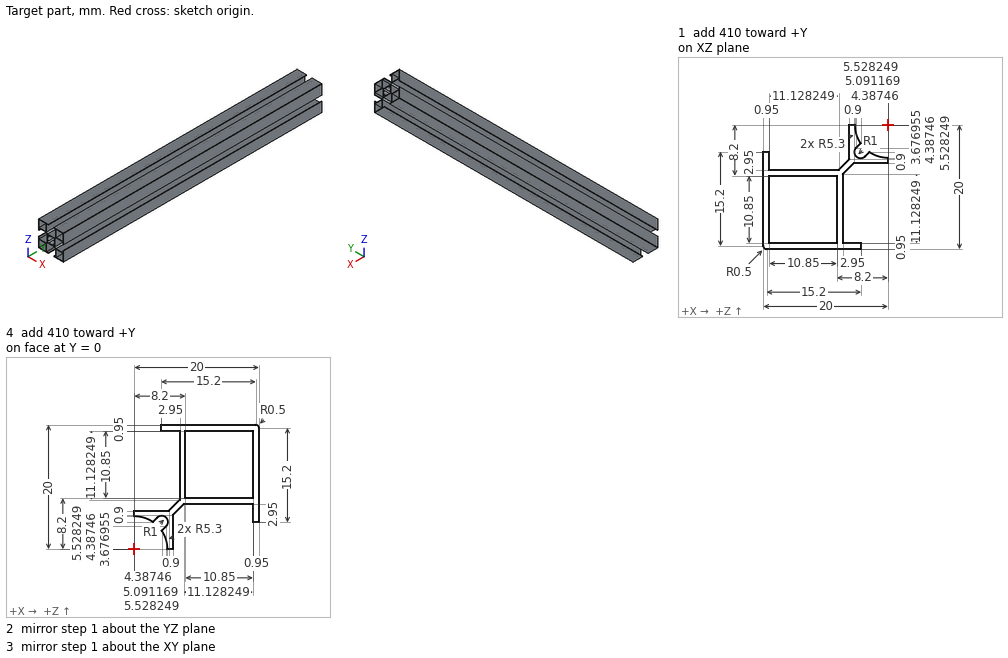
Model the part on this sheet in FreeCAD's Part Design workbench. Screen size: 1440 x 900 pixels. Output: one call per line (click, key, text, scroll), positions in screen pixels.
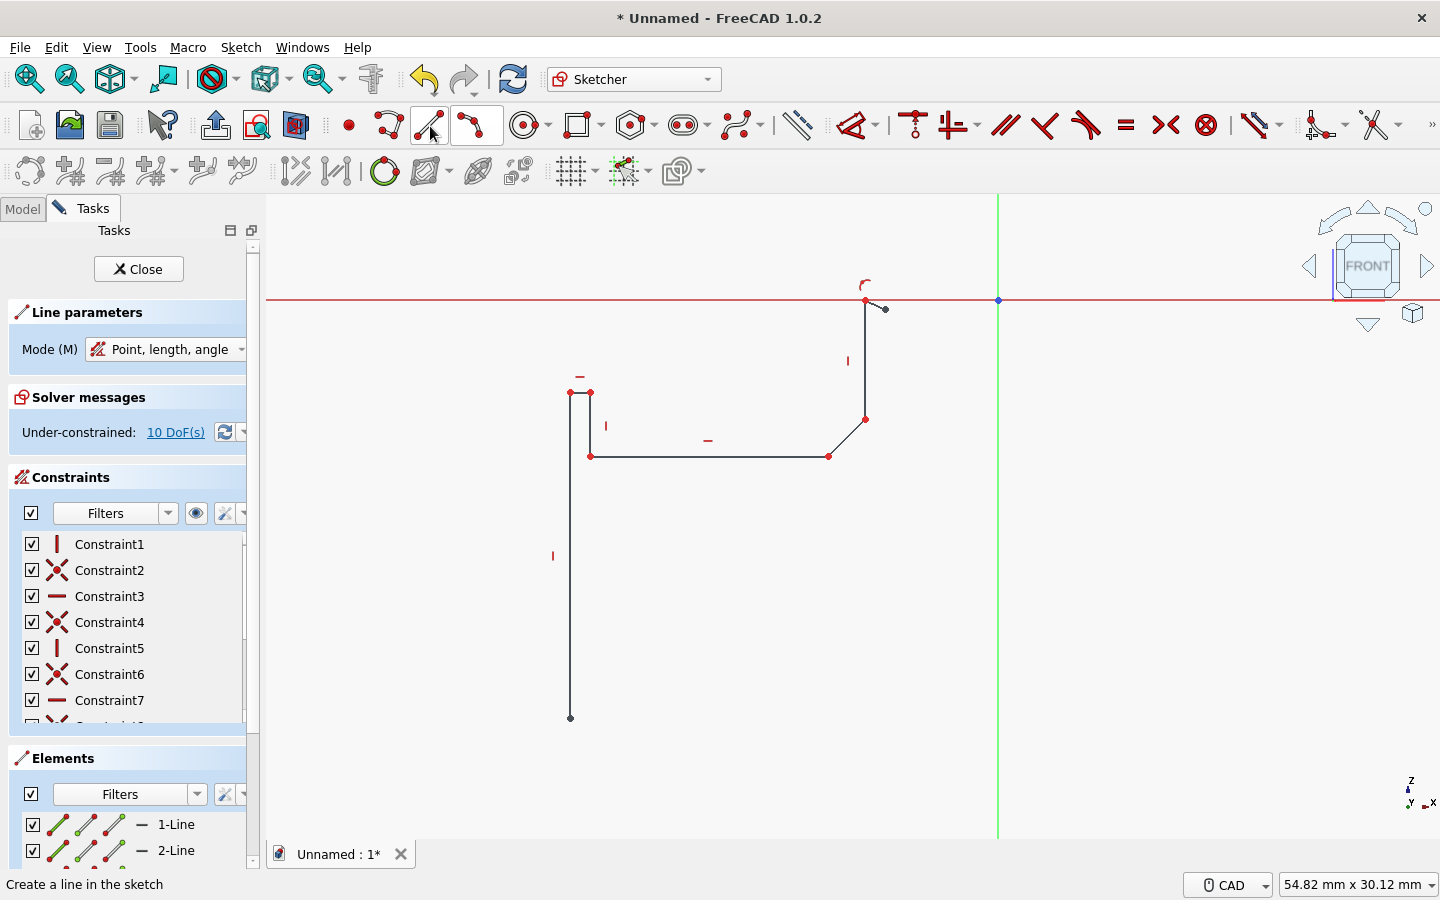
click(904, 364)
click(889, 379)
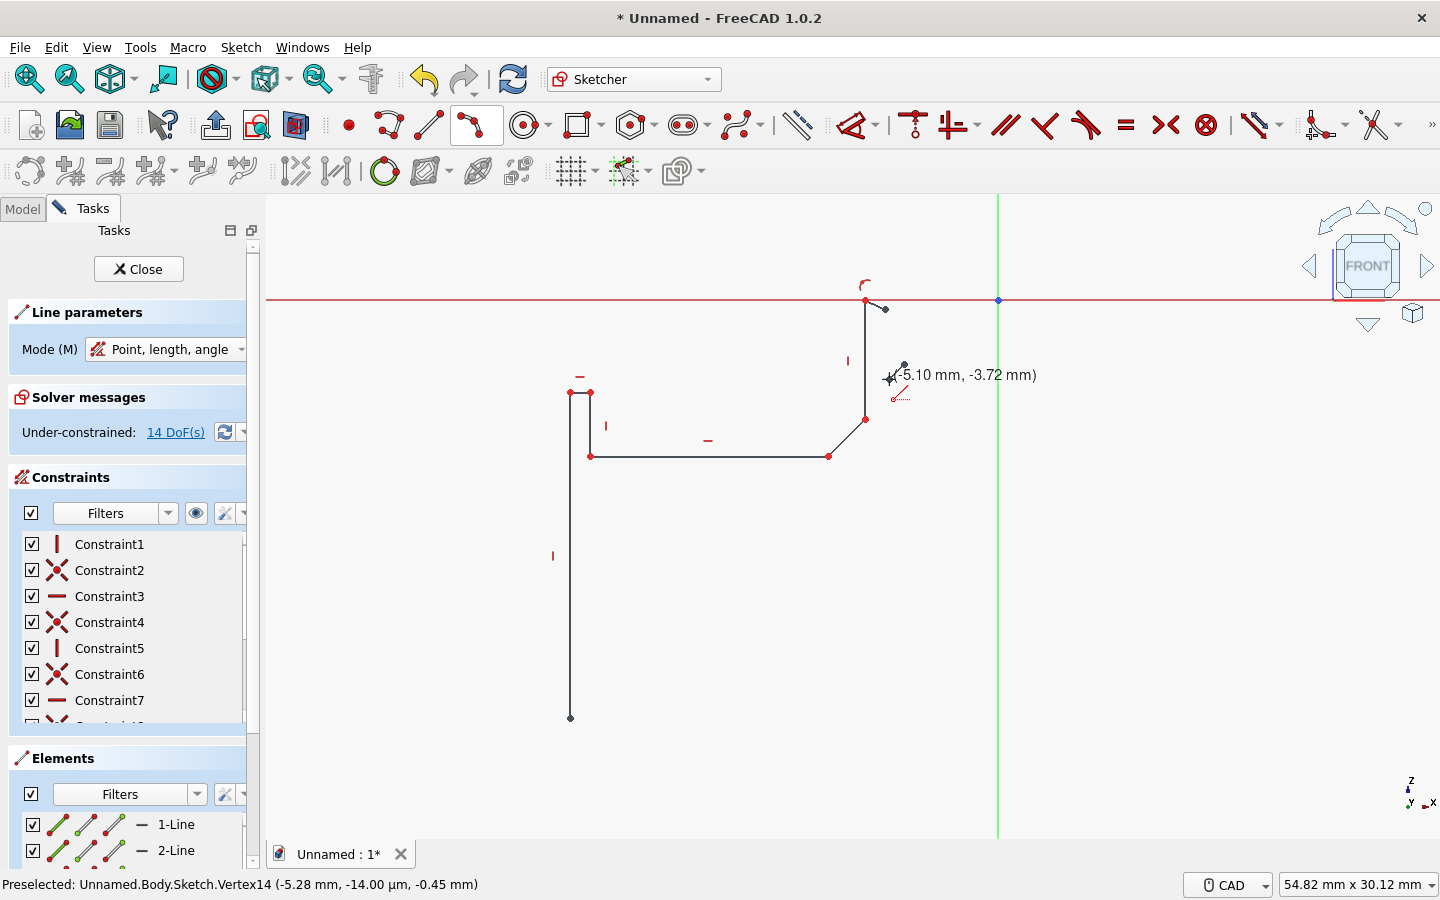
click(919, 409)
click(934, 394)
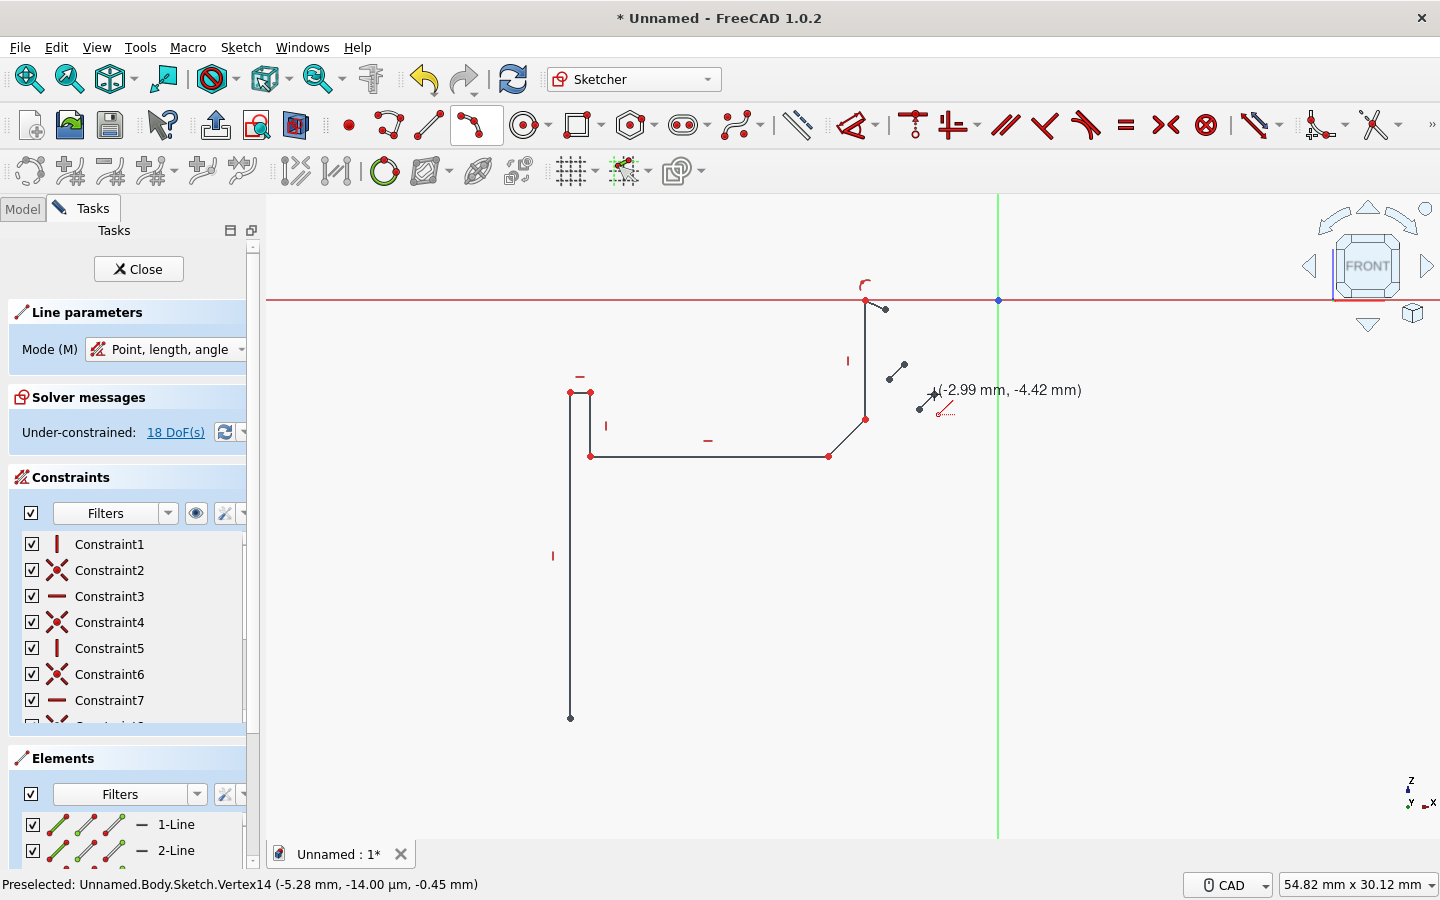
click(390, 126)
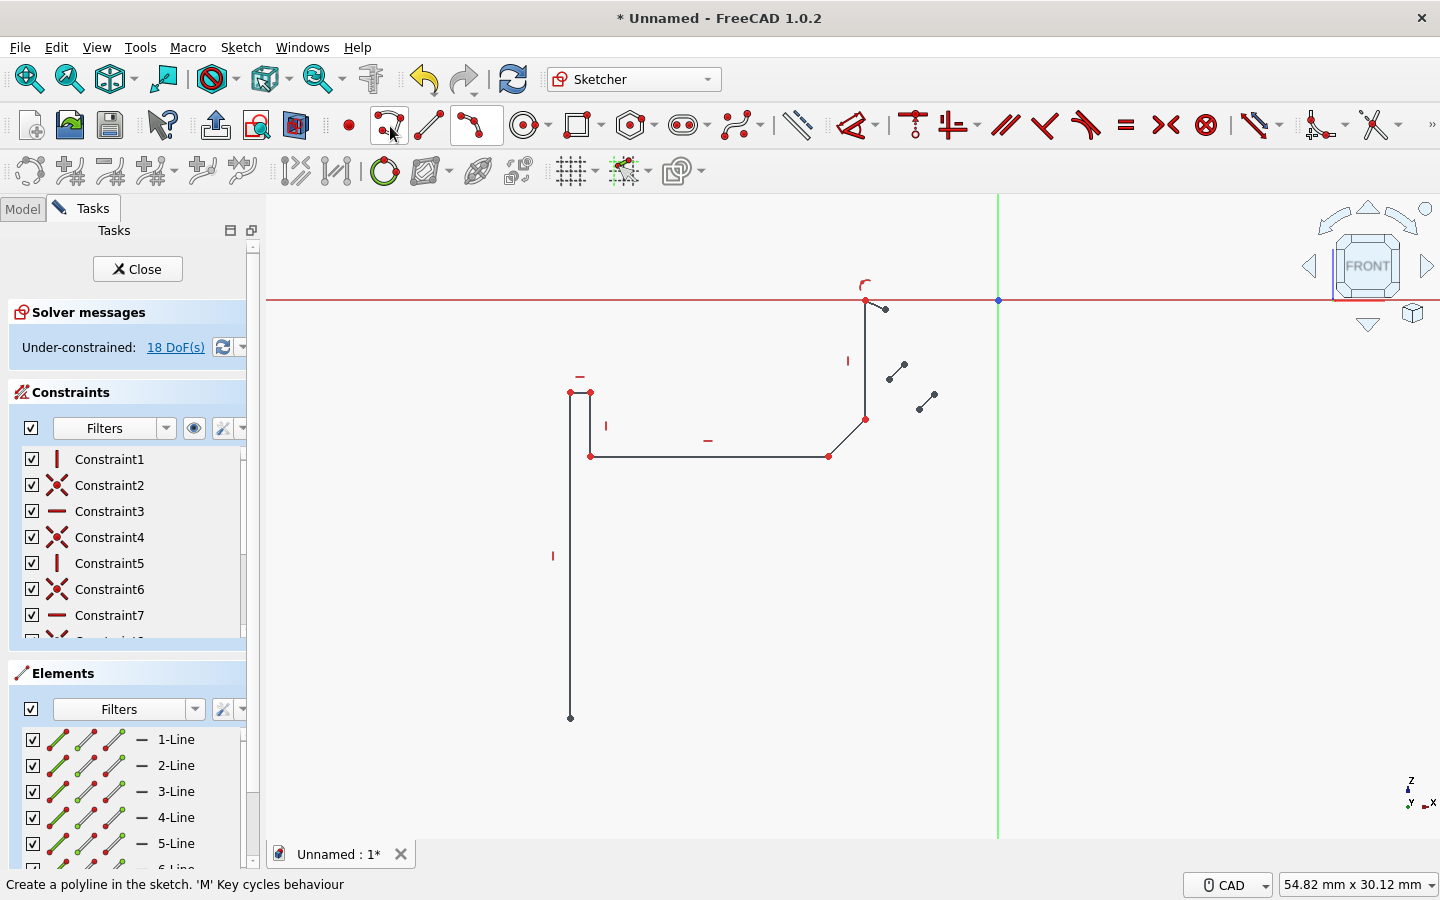
click(998, 414)
click(989, 433)
click(880, 433)
click(843, 470)
click(843, 708)
click(906, 708)
click(906, 729)
click(581, 729)
right_click(581, 729)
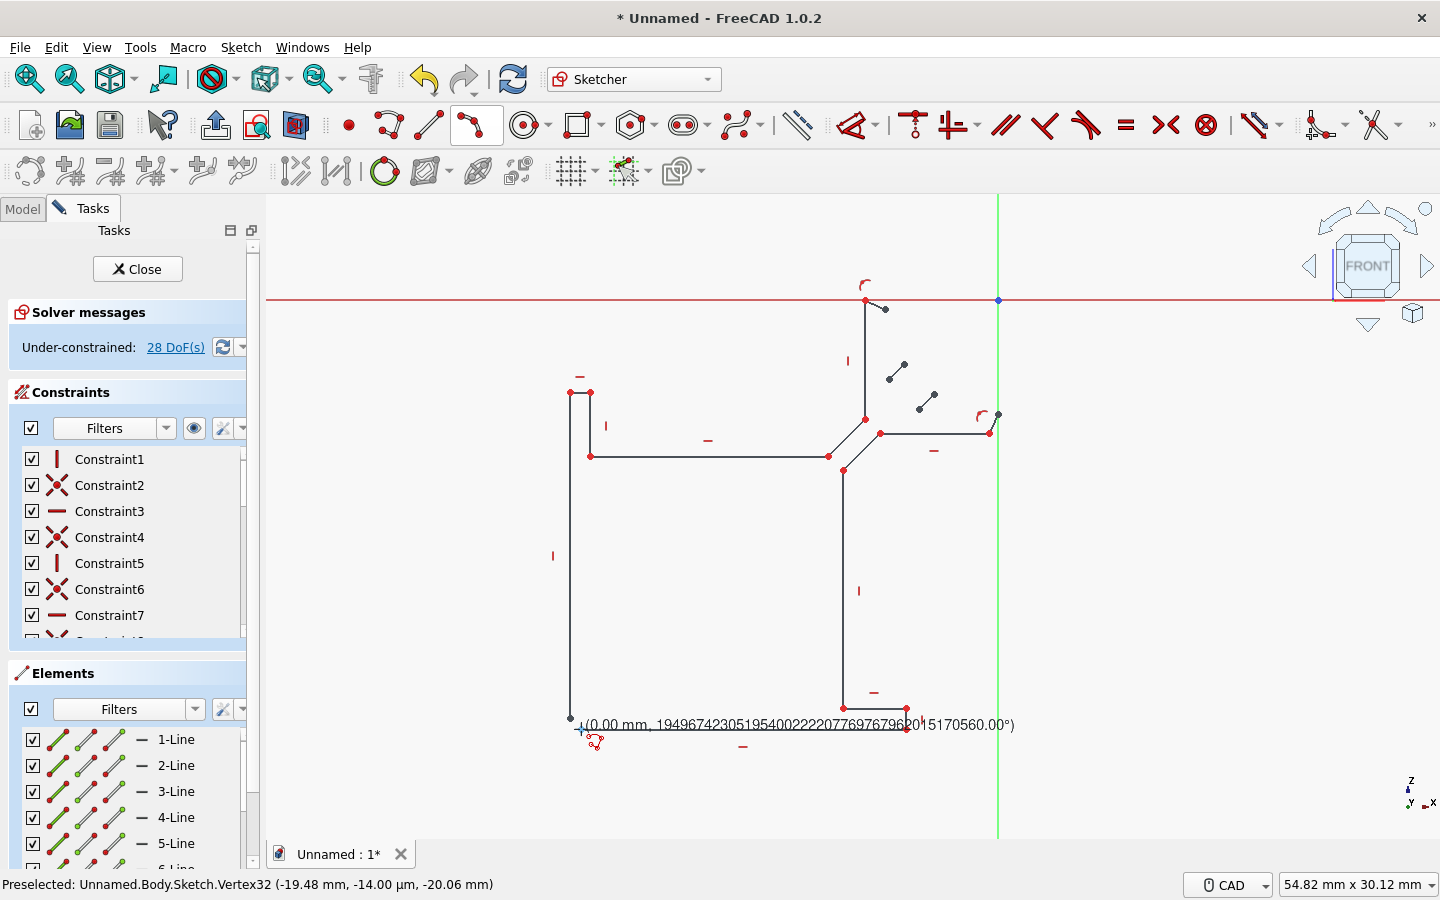
click(470, 126)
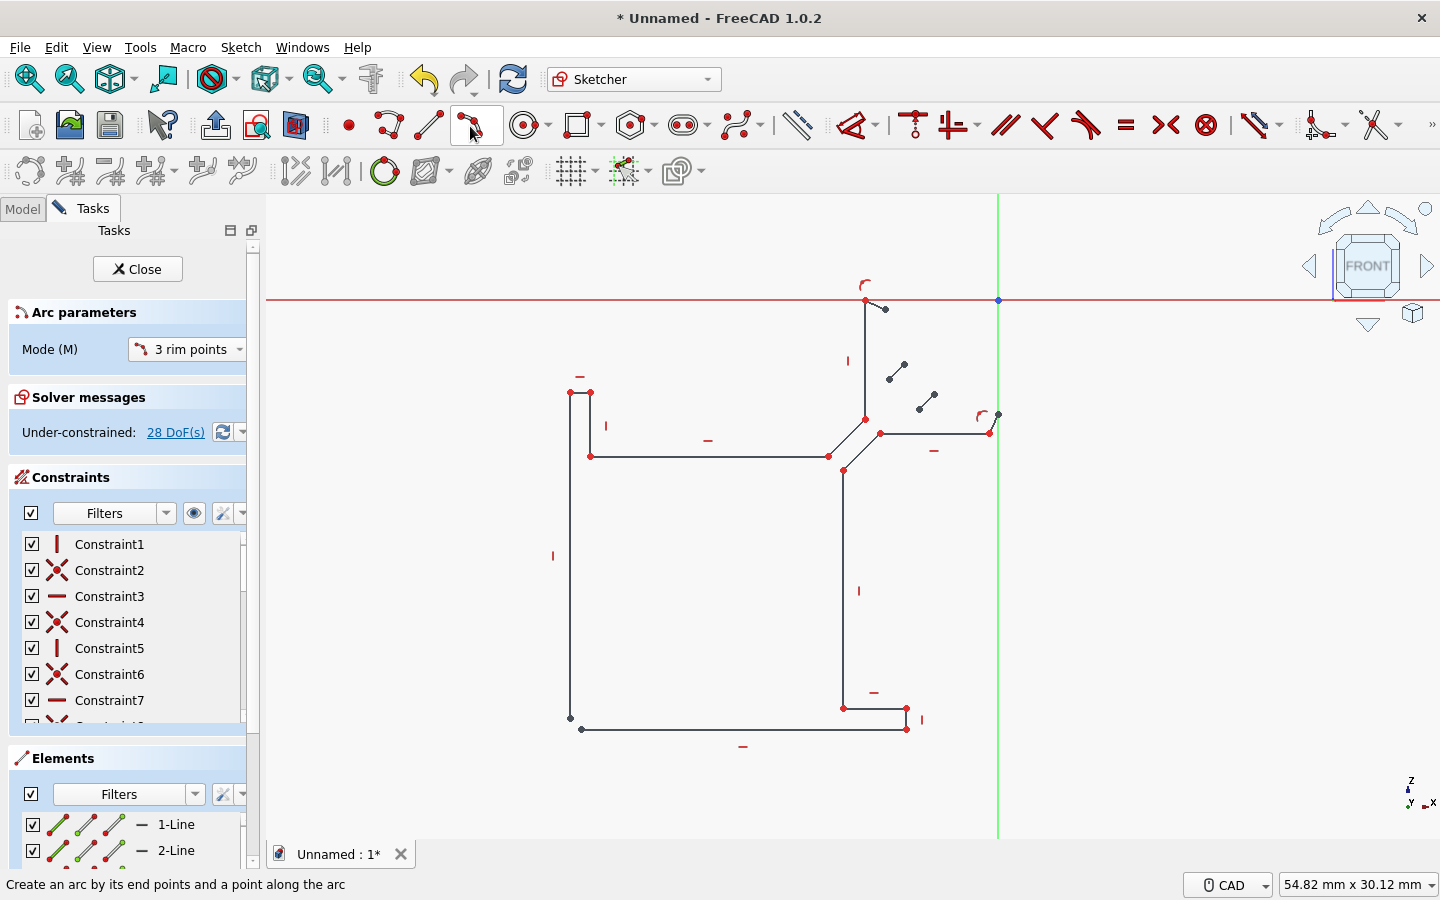
scroll(885, 300, up, 3)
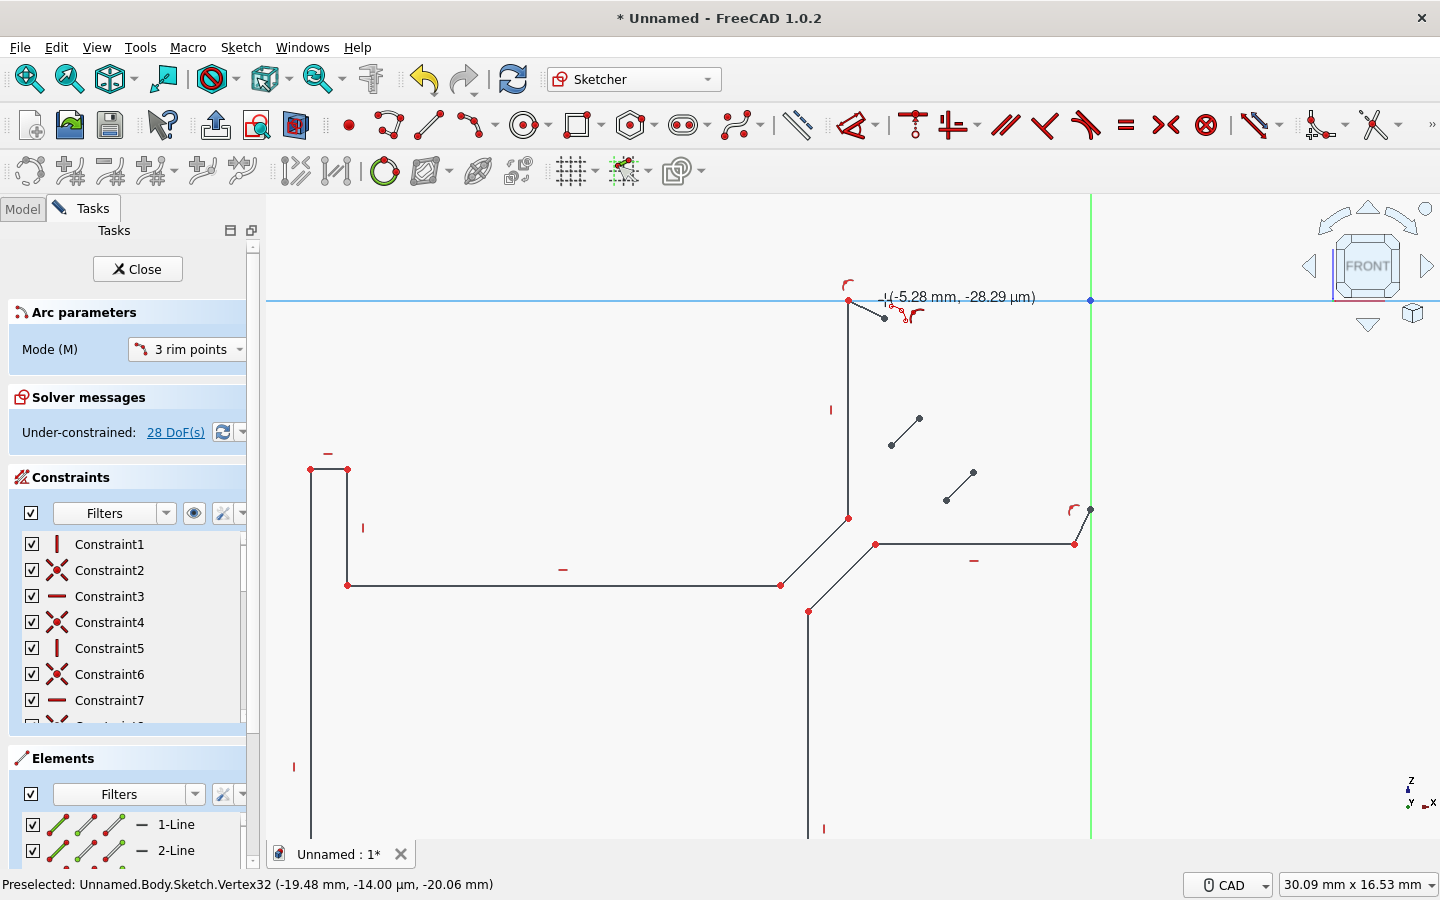
click(885, 318)
click(919, 418)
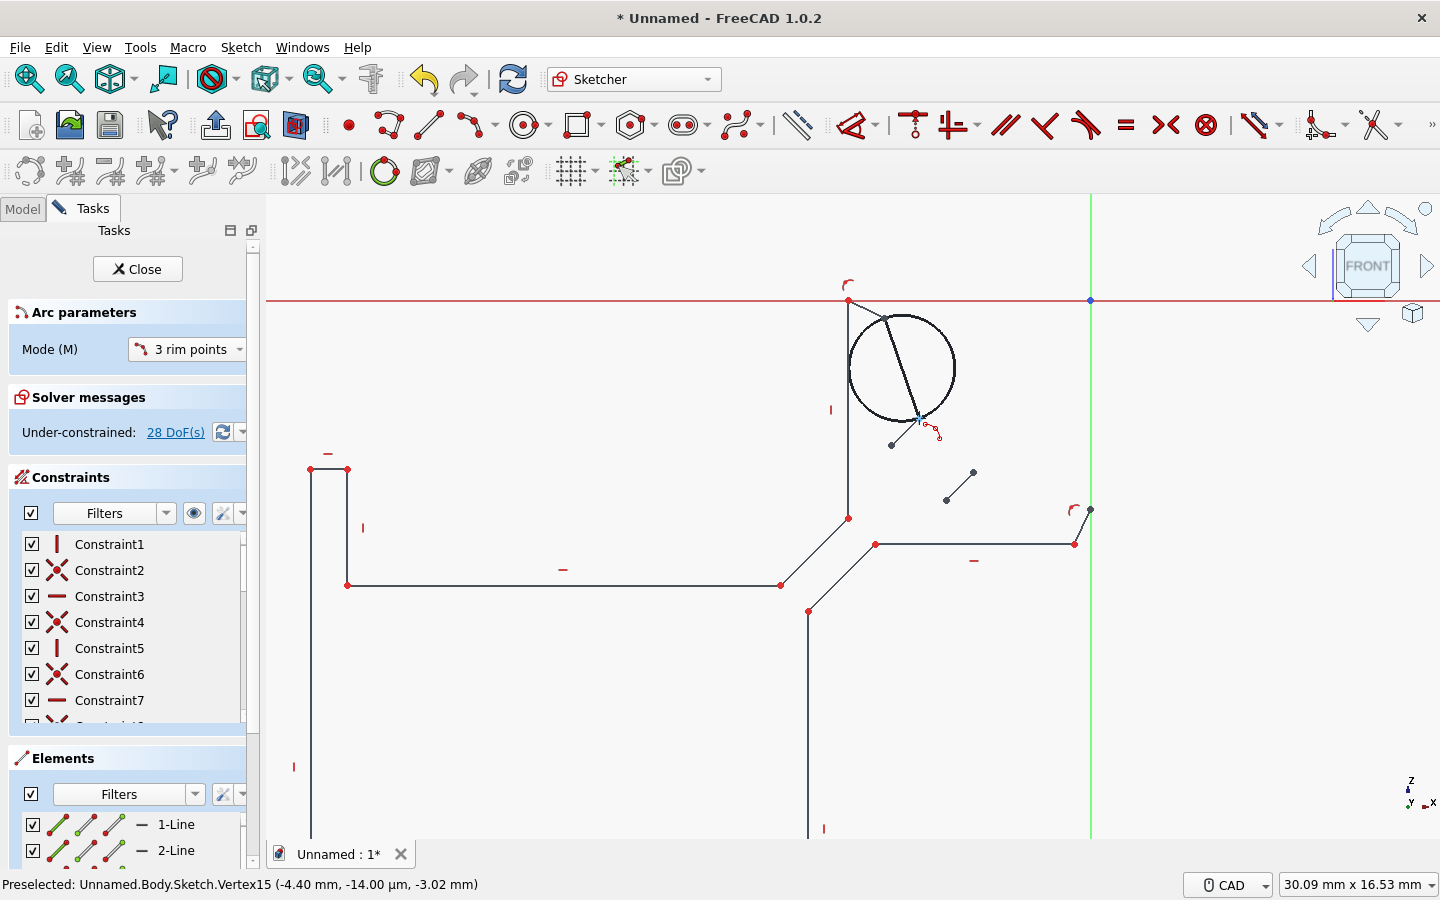
scroll(893, 361, up, 3)